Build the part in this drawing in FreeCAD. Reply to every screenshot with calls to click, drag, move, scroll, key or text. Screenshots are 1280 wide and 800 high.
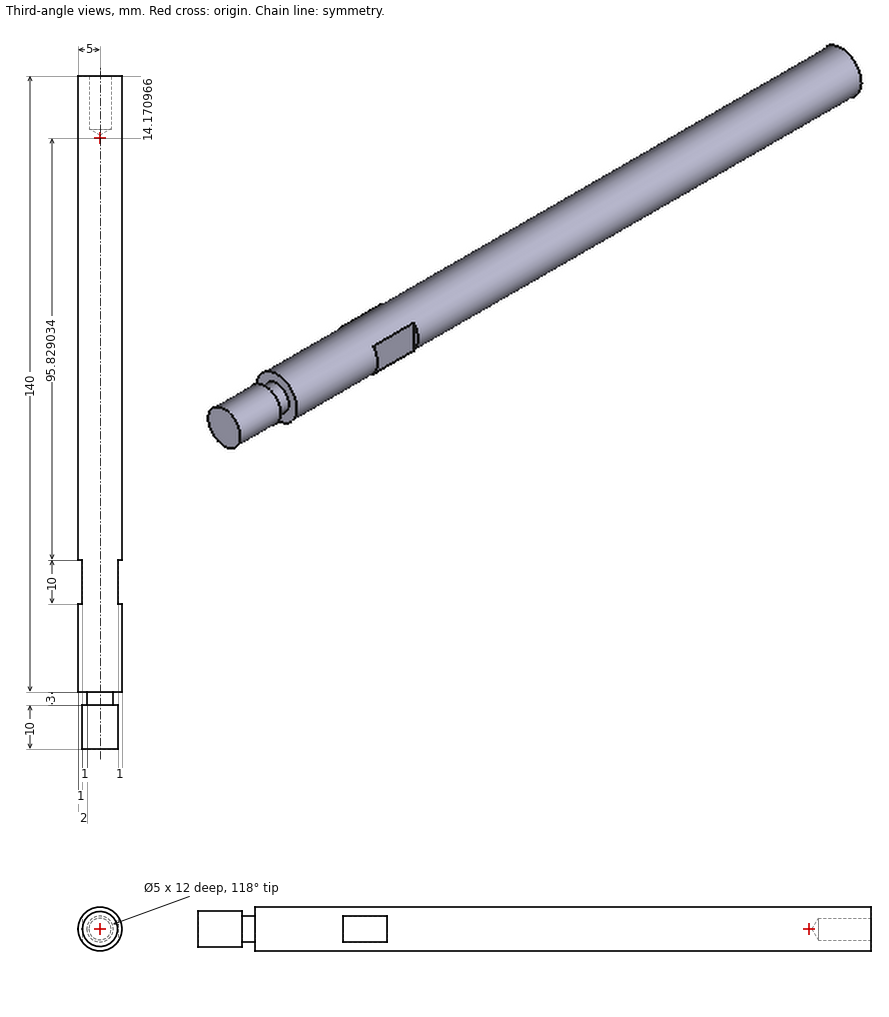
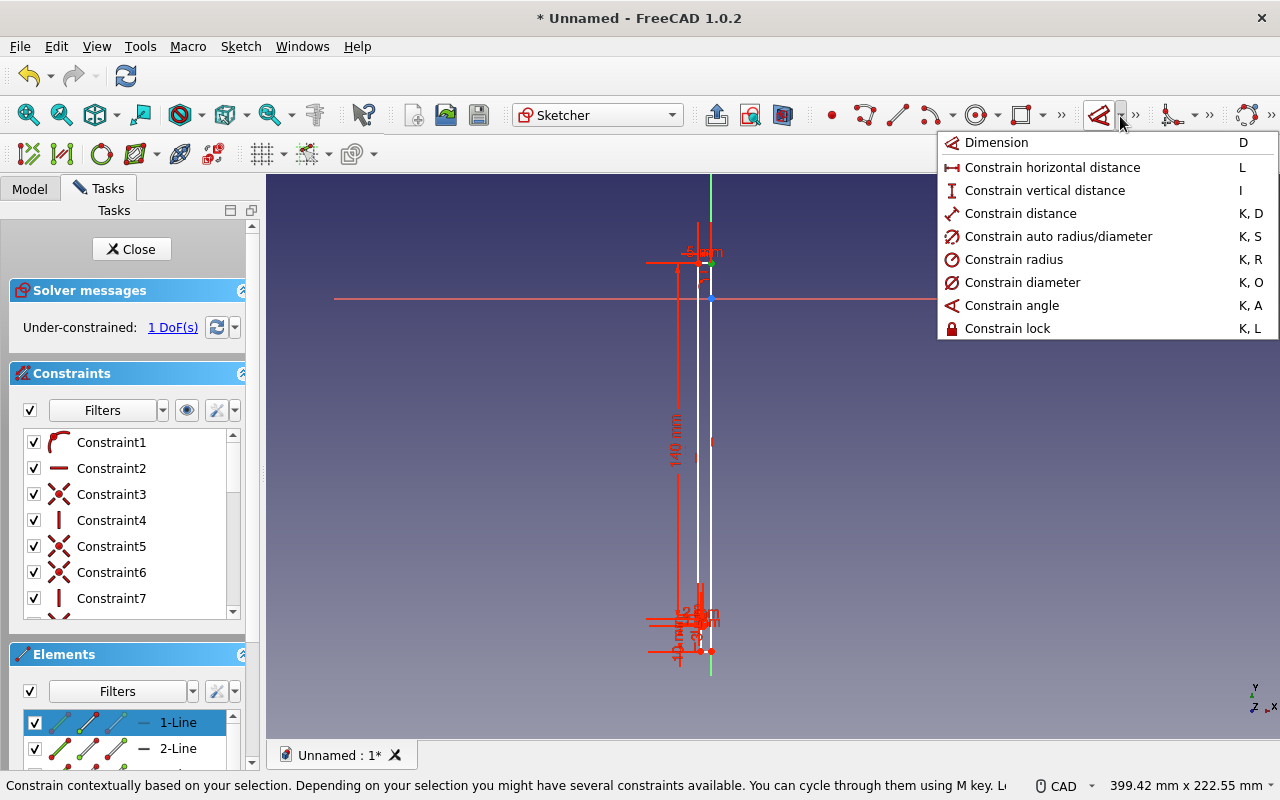
click(1108, 190)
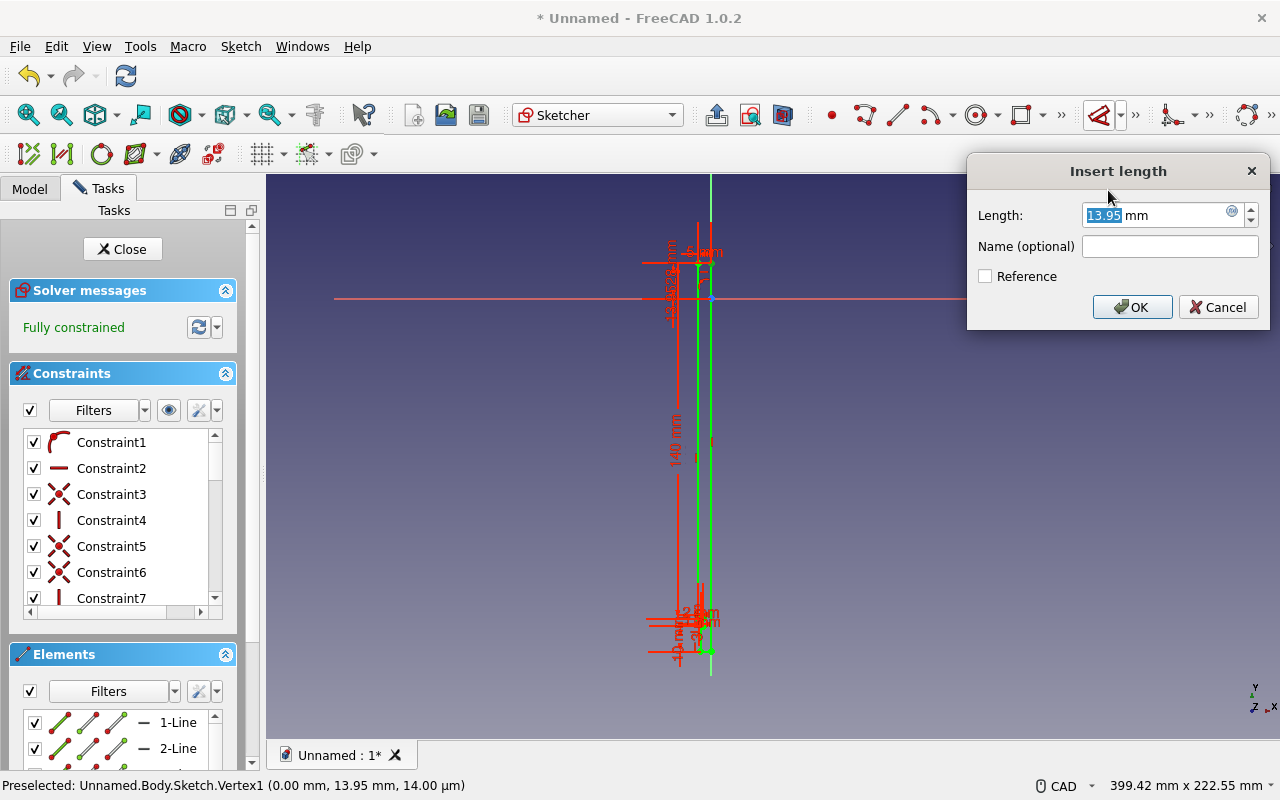
text(14.170966)
key(Return)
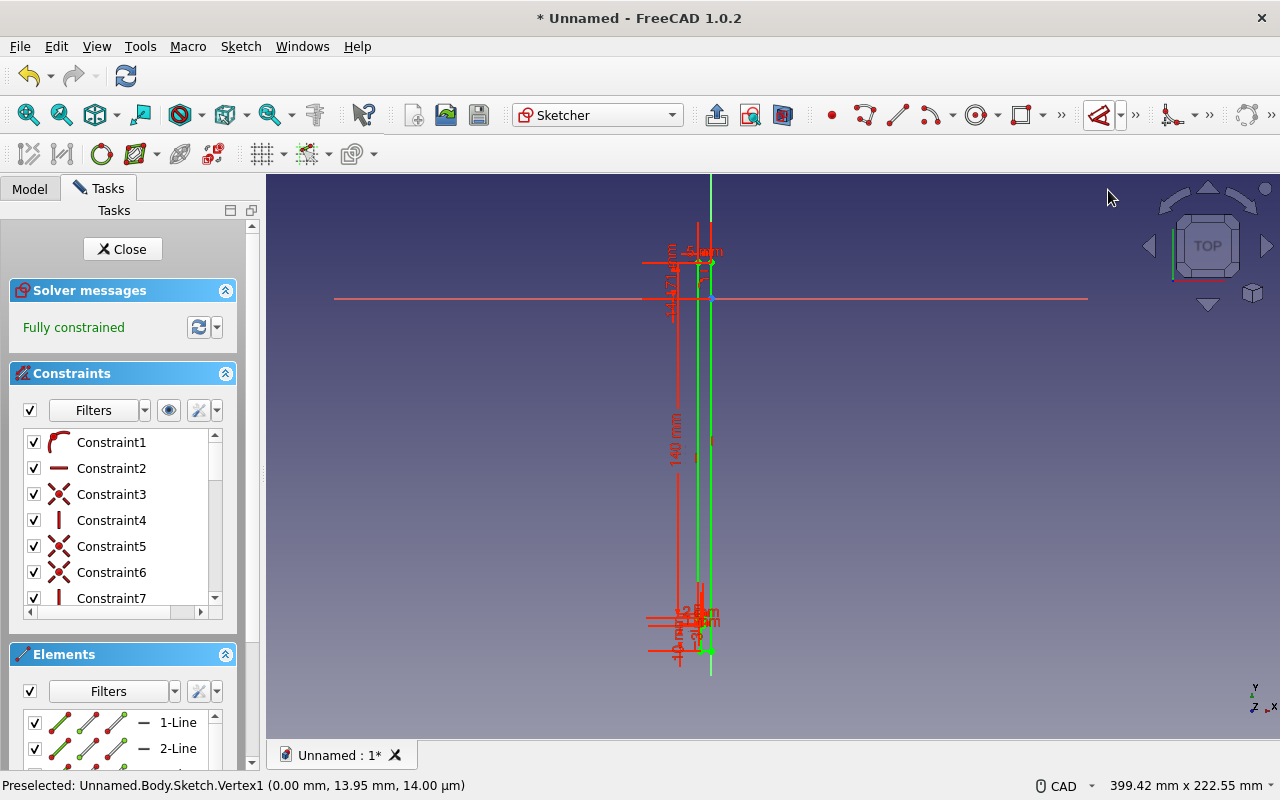
click(123, 249)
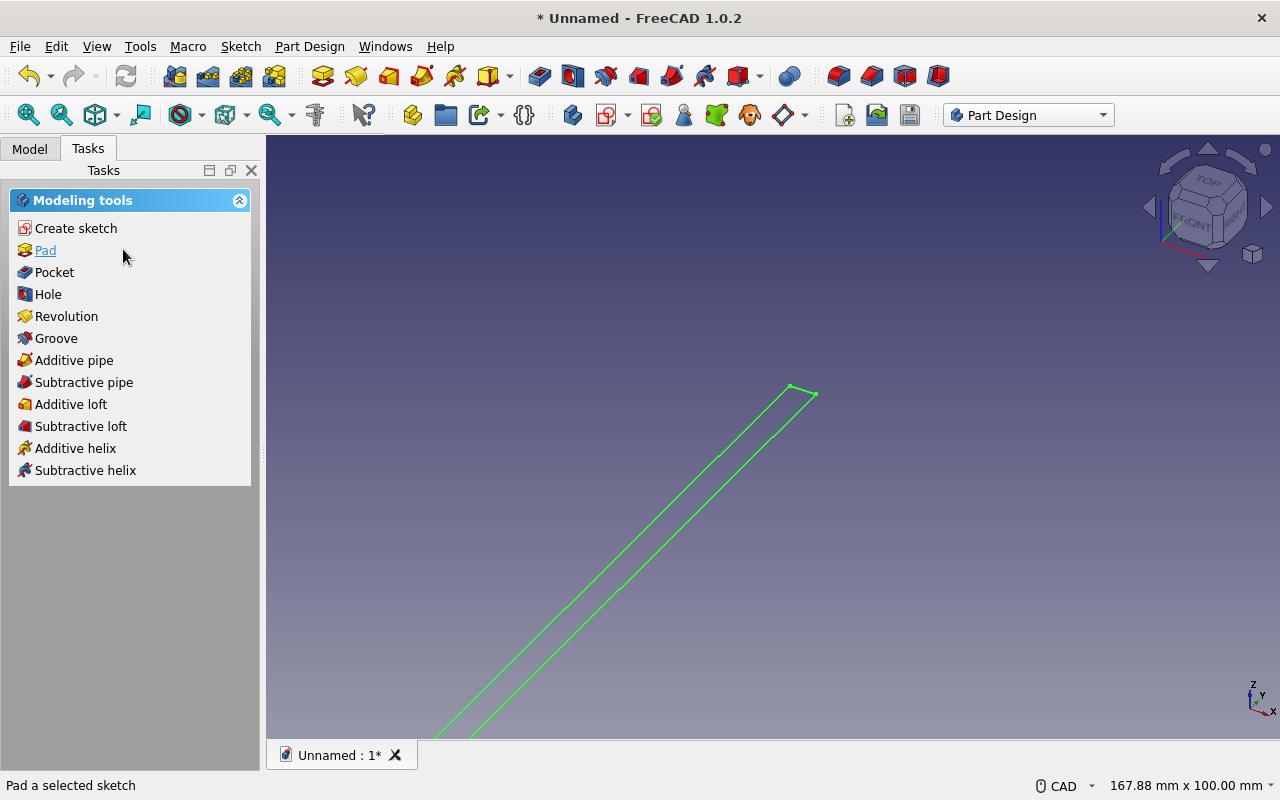
click(356, 76)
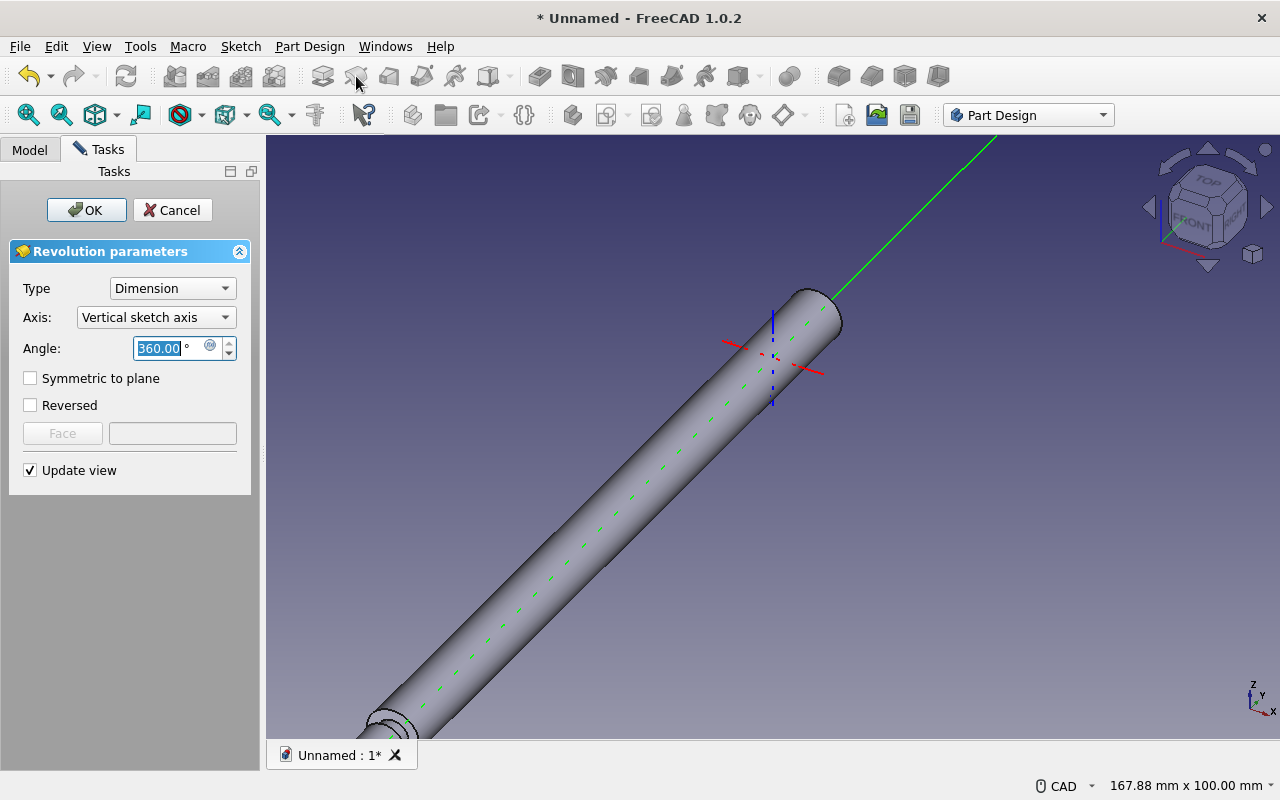
click(87, 210)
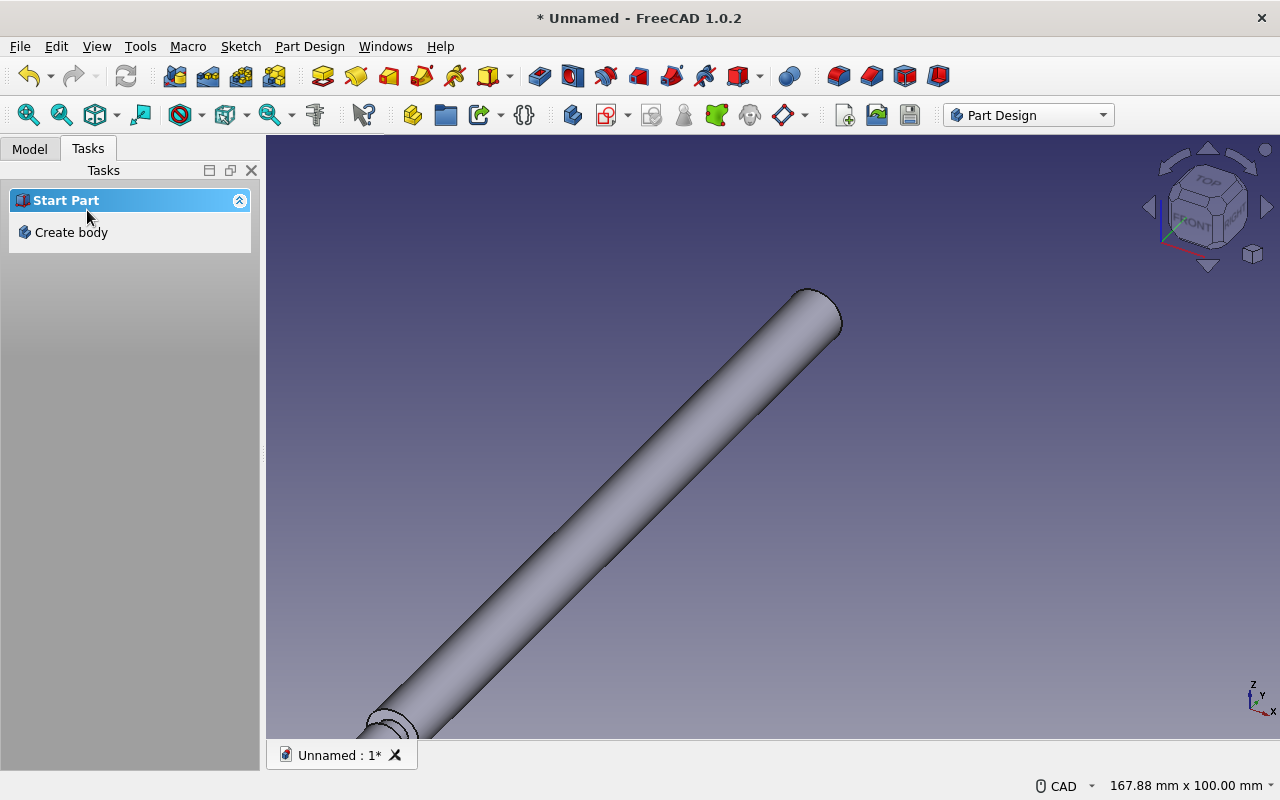
click(29, 116)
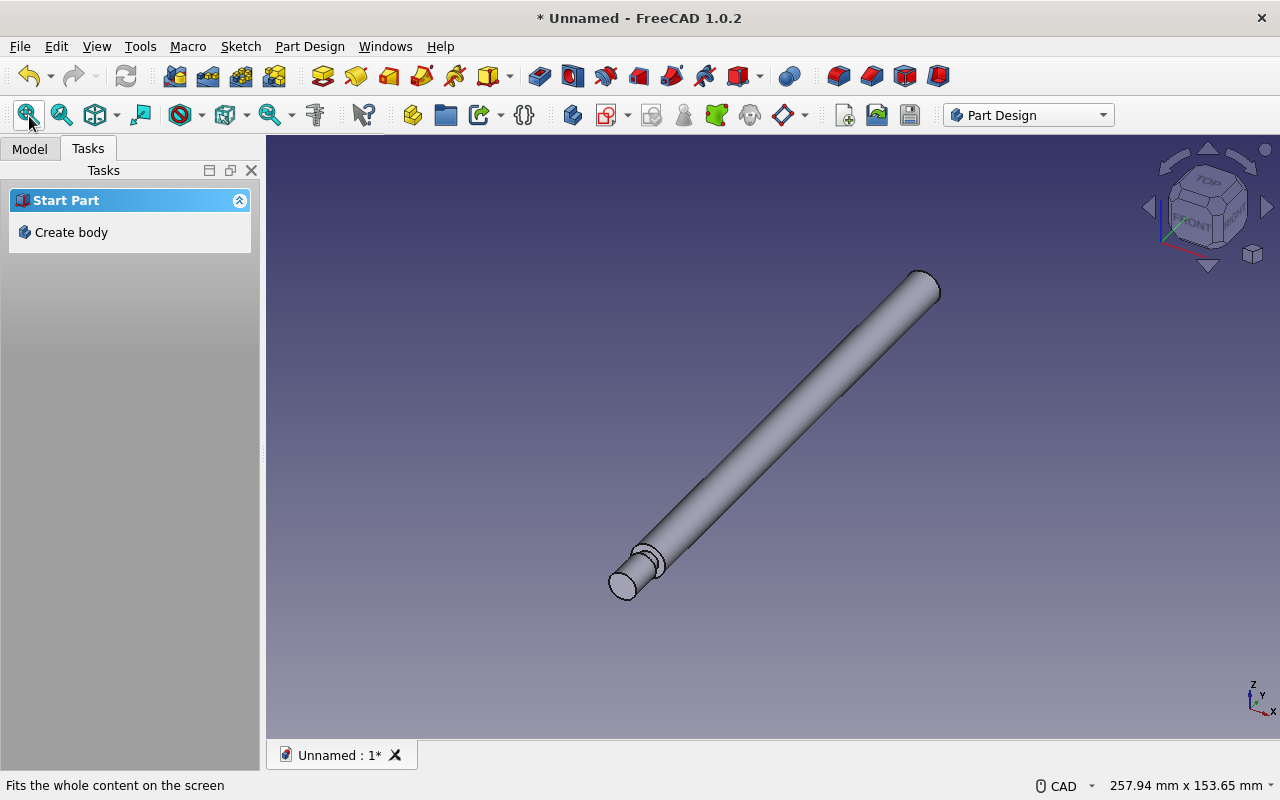
click(606, 116)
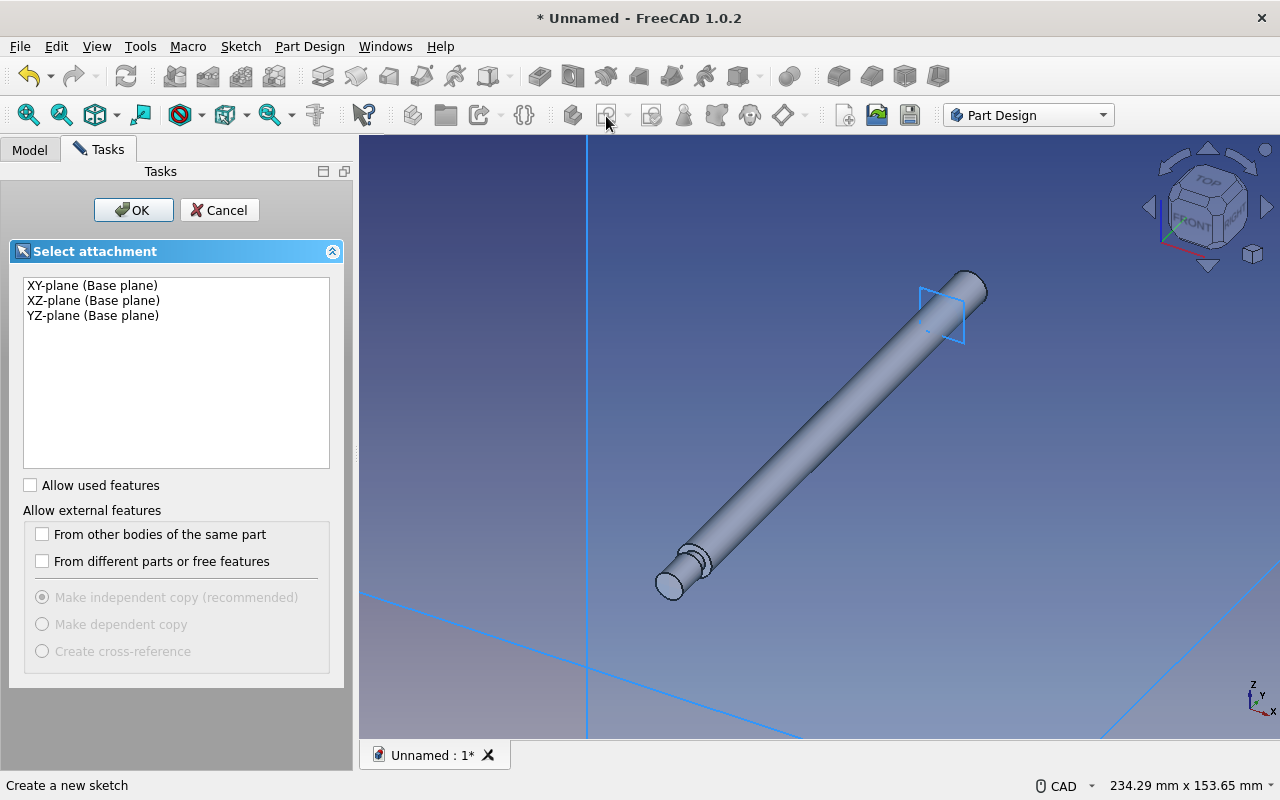
click(84, 286)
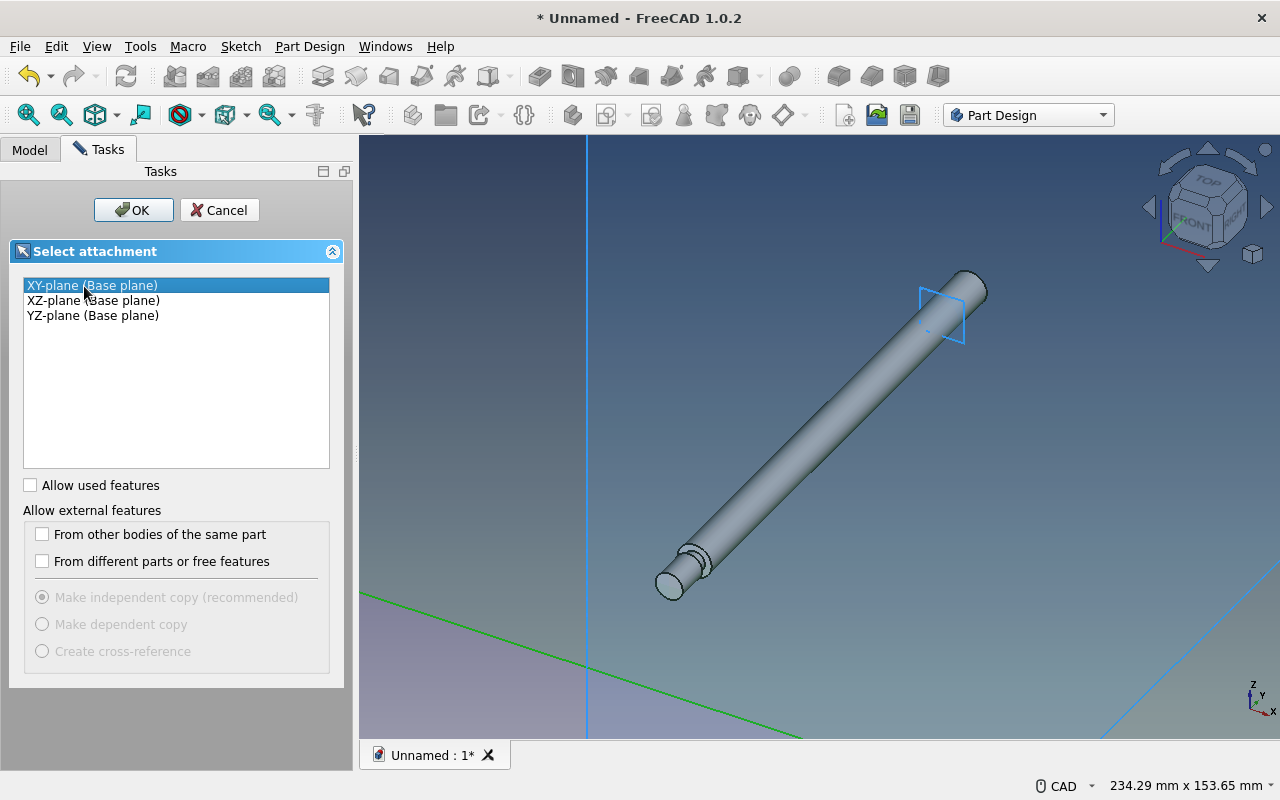
click(134, 210)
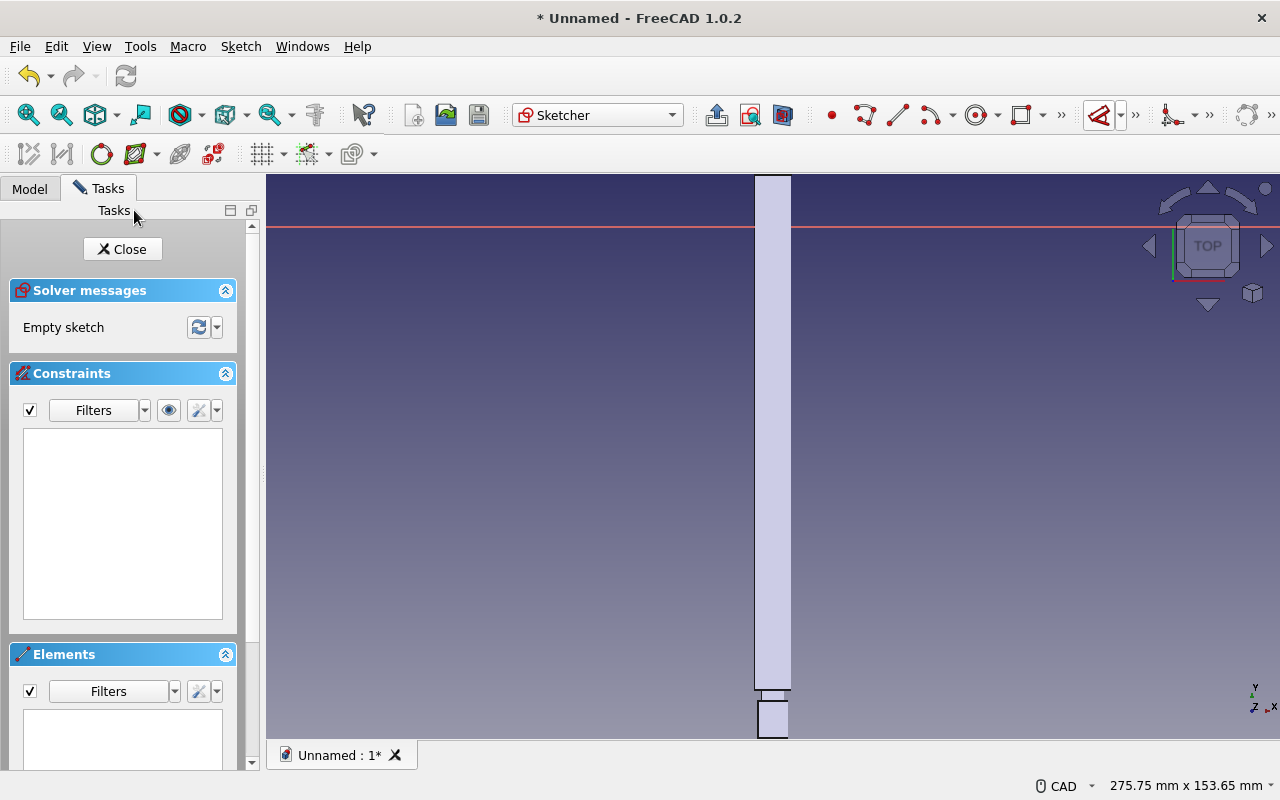
click(783, 116)